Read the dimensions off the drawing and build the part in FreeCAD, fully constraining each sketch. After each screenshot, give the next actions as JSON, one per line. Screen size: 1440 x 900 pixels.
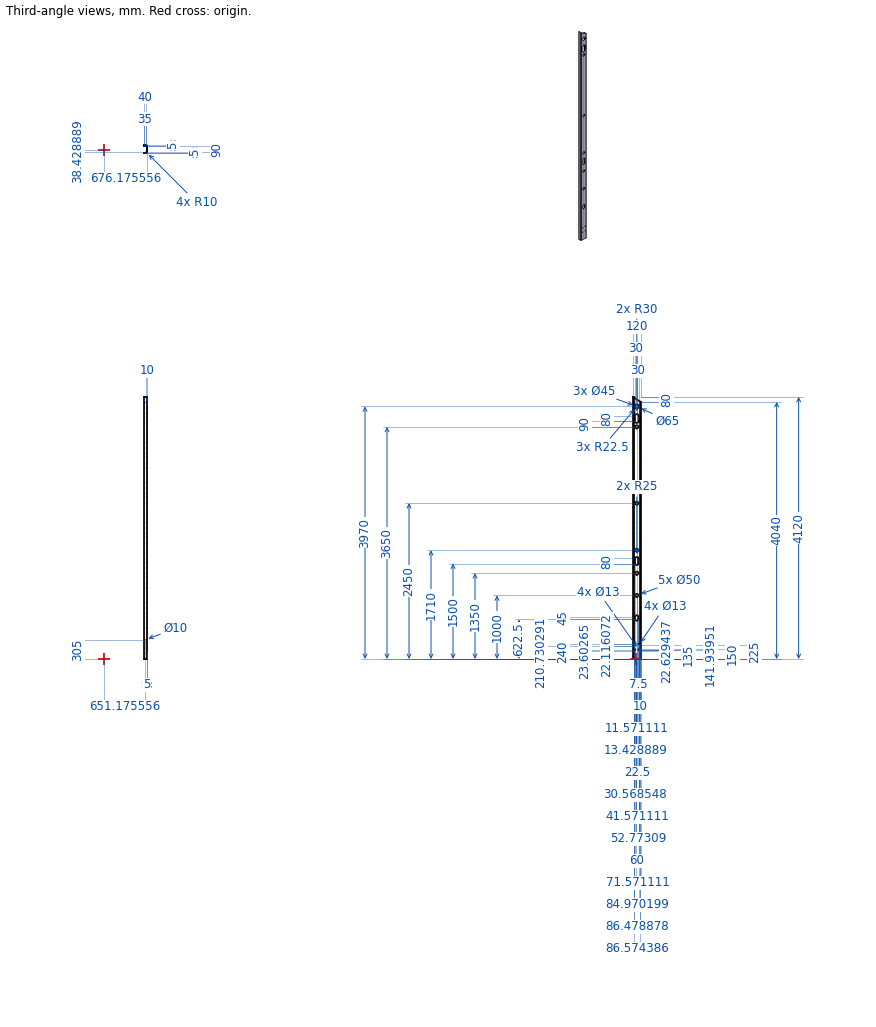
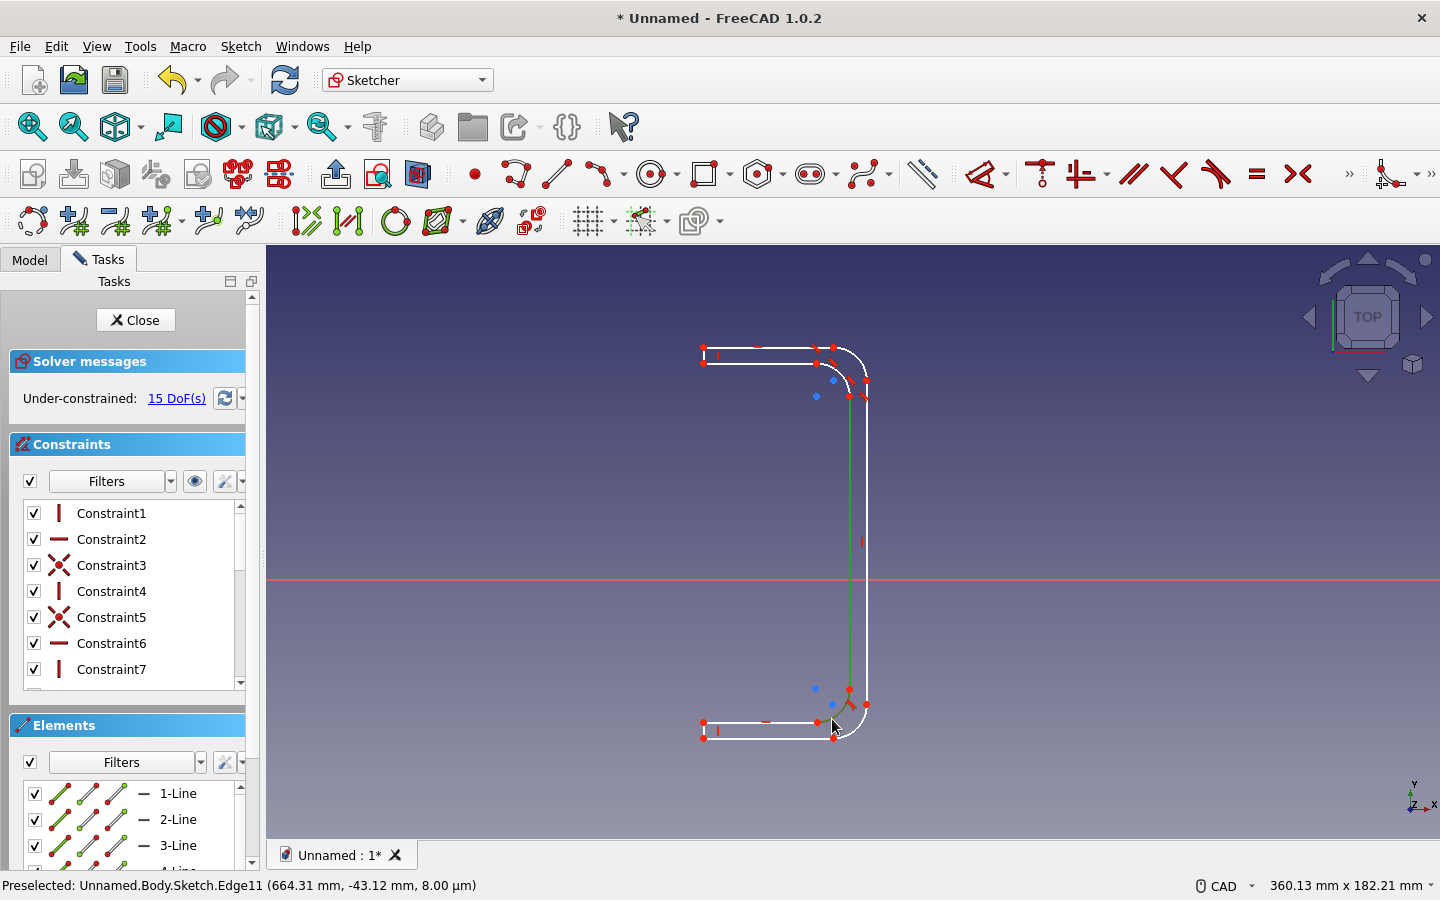
{"action": "left_click", "coordinate": [1216, 174]}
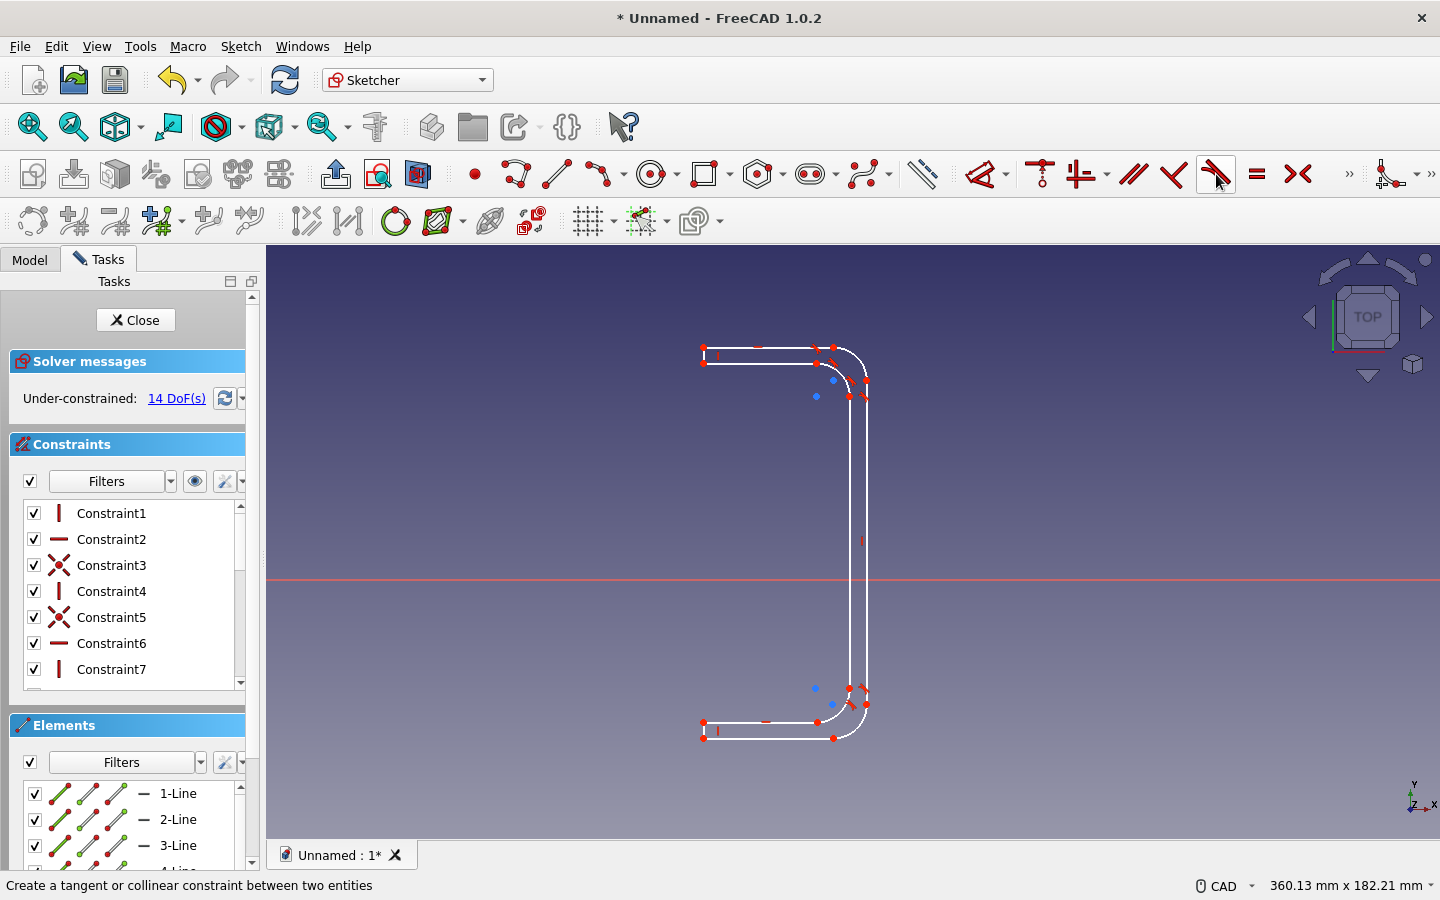
{"action": "left_click", "coordinate": [784, 723]}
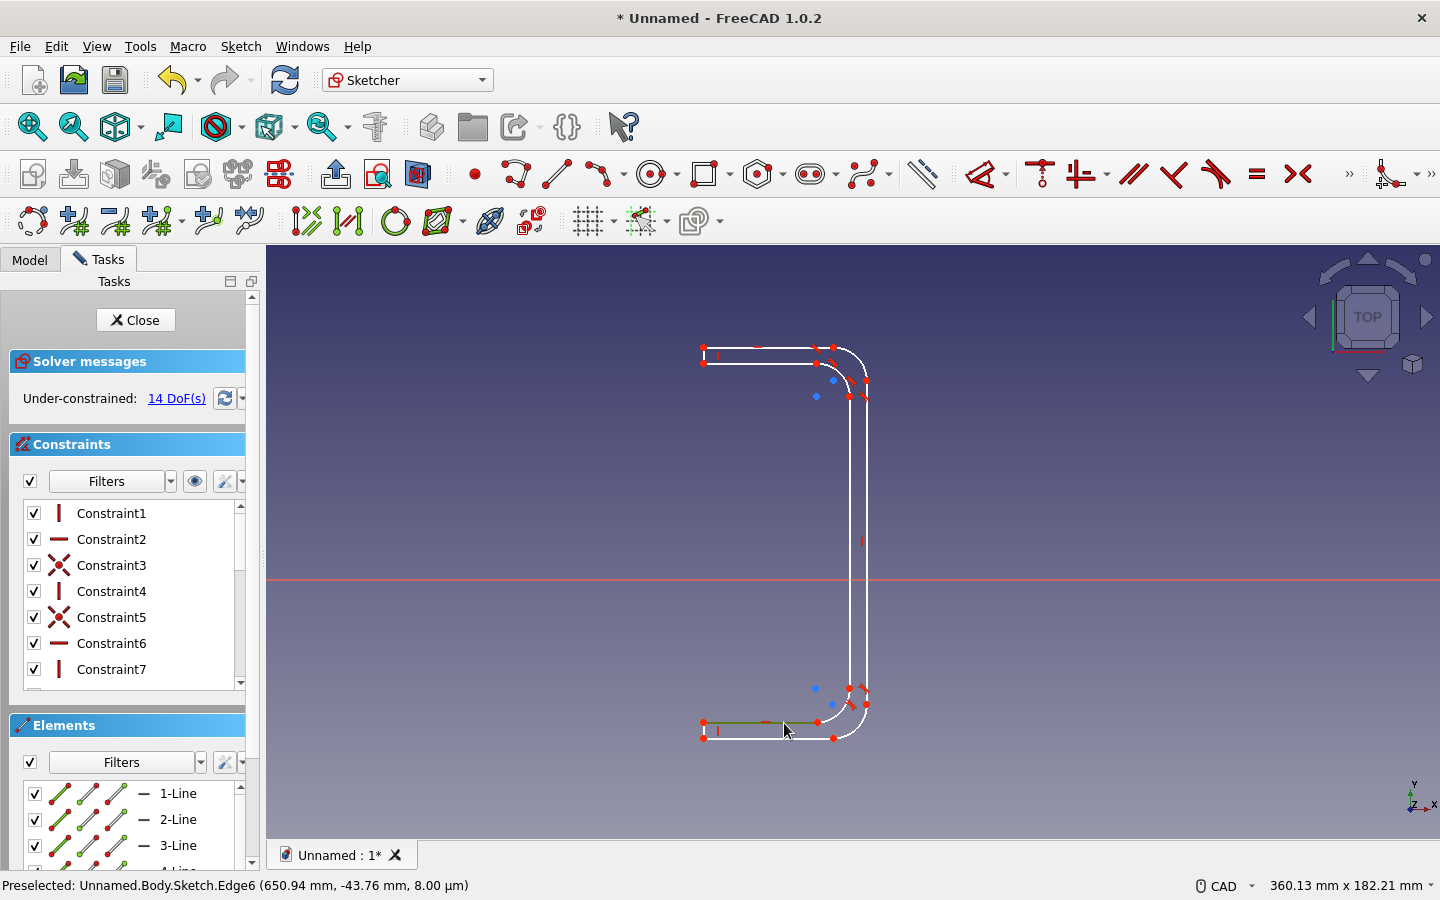
{"action": "left_click", "coordinate": [832, 718]}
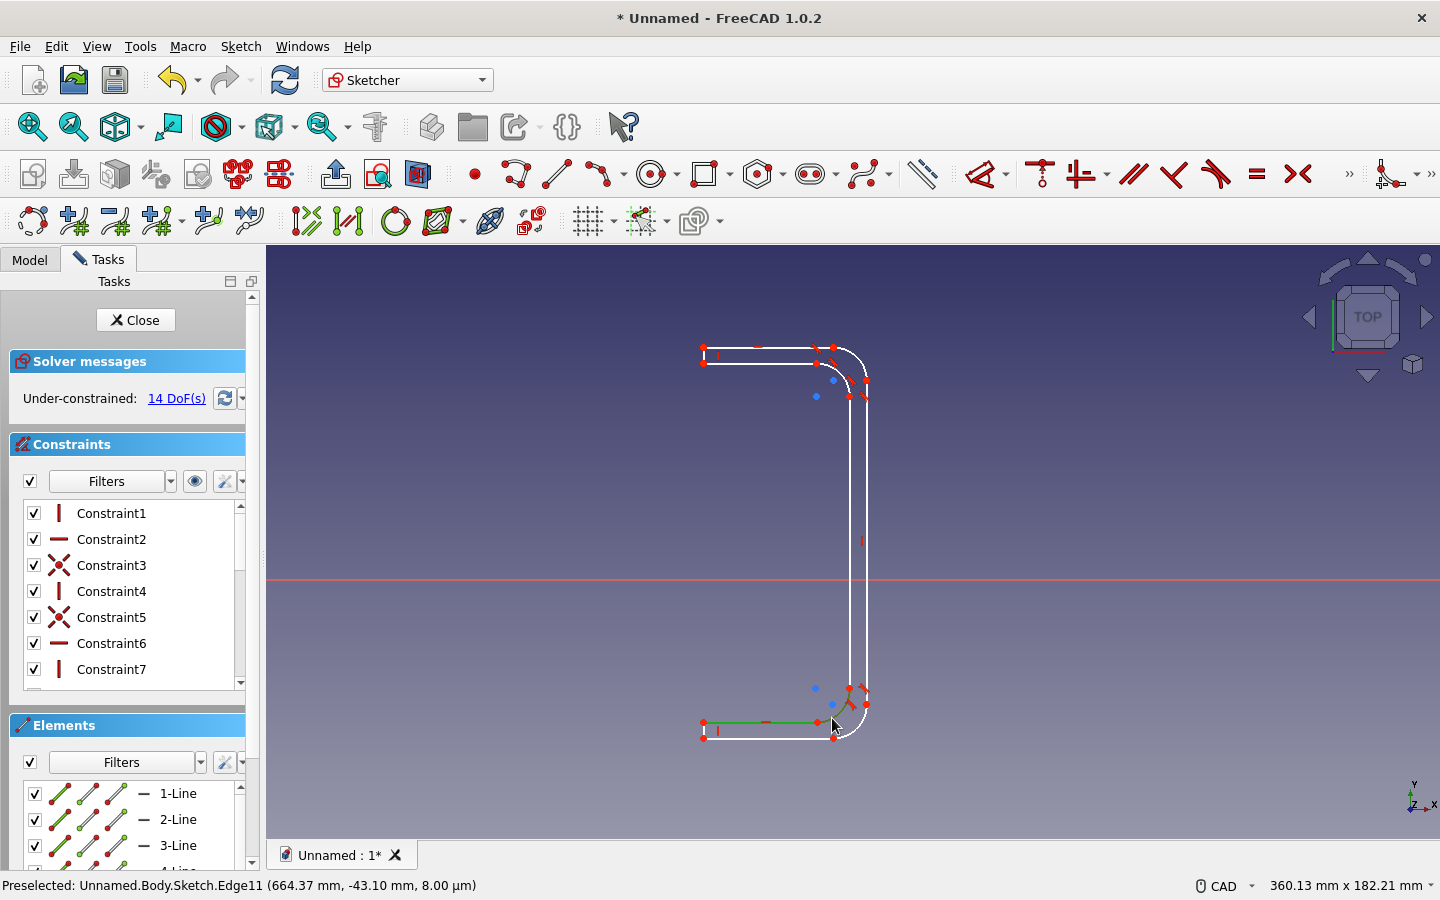
{"action": "key", "text": "t"}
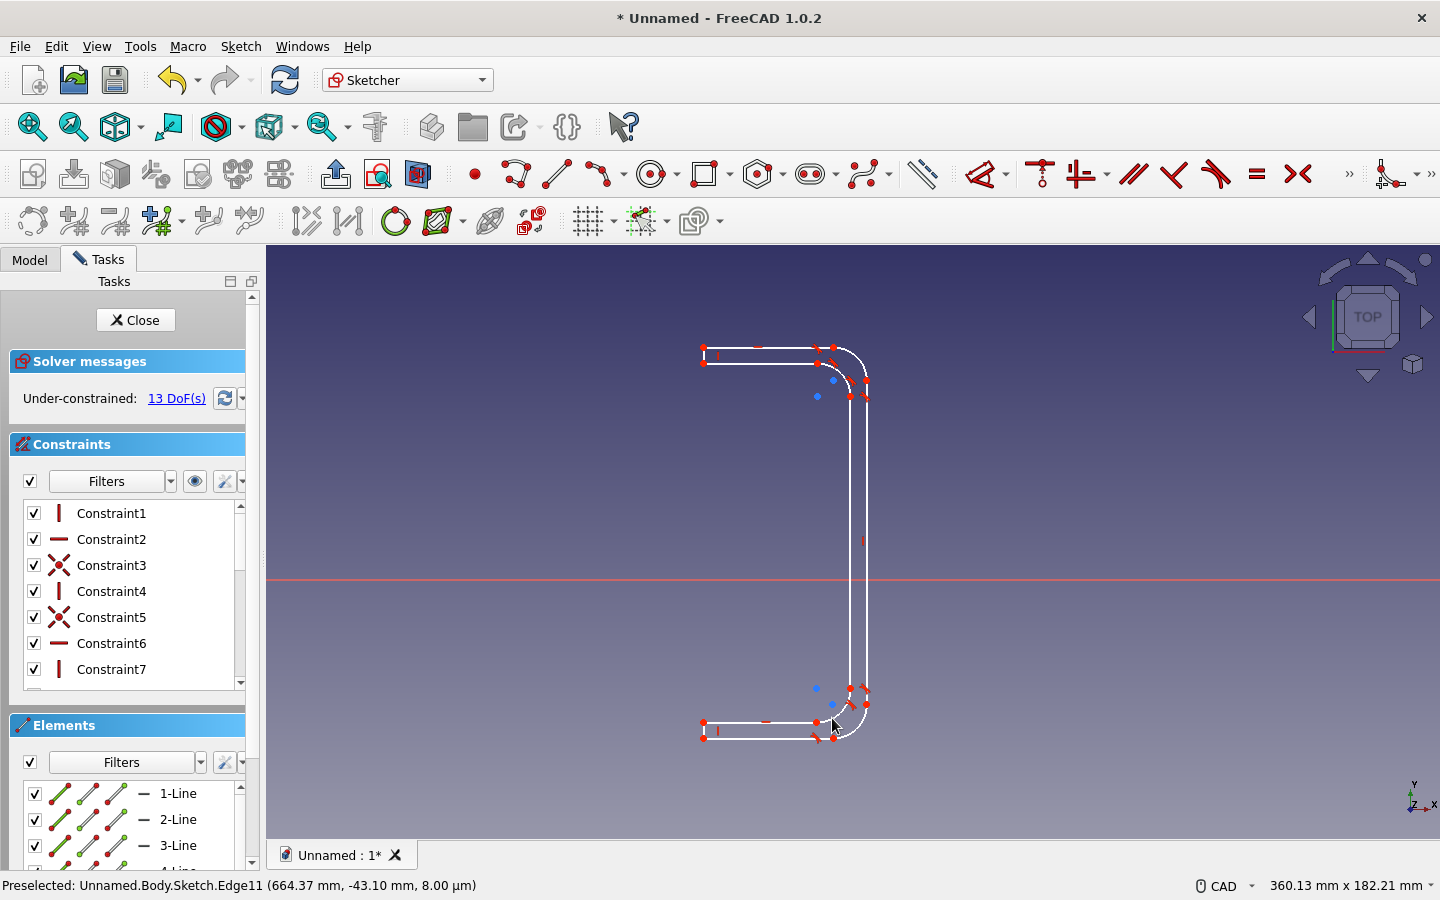
{"action": "left_click", "coordinate": [743, 739]}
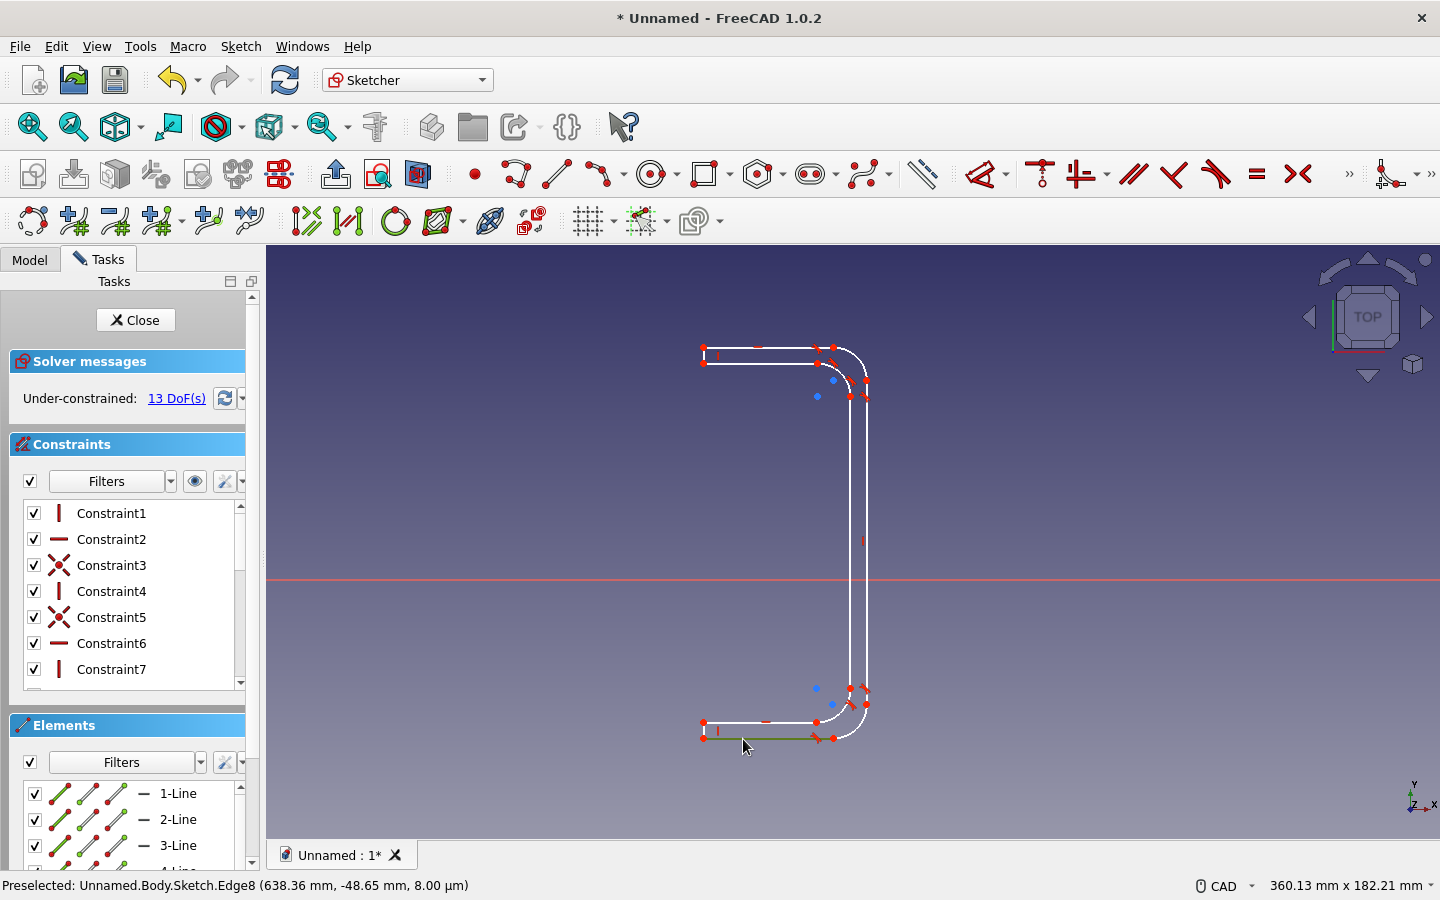
{"action": "left_click", "coordinate": [849, 735]}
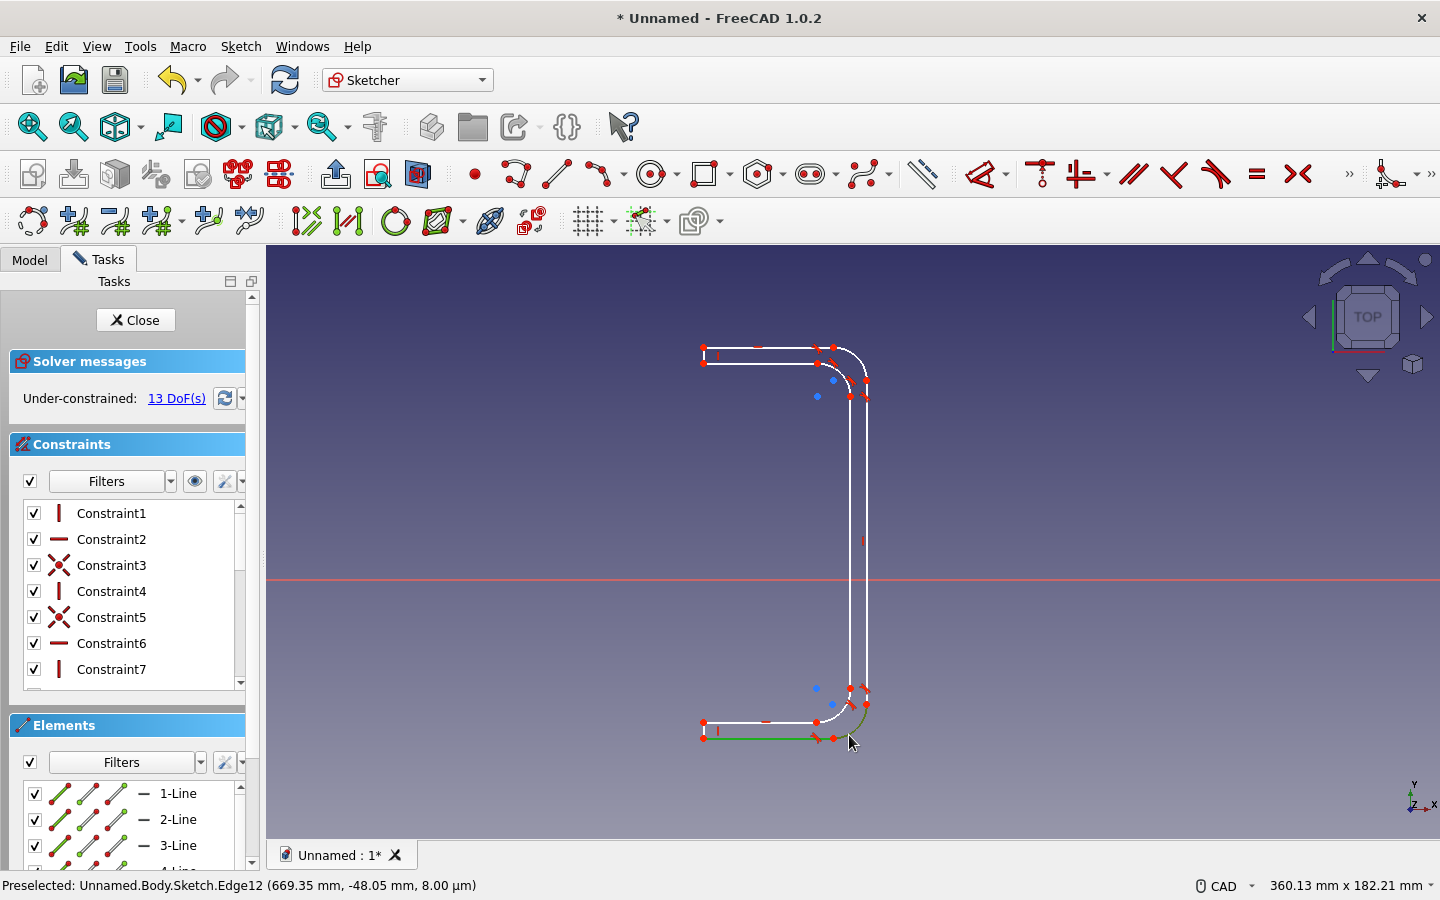
{"action": "key", "text": "t"}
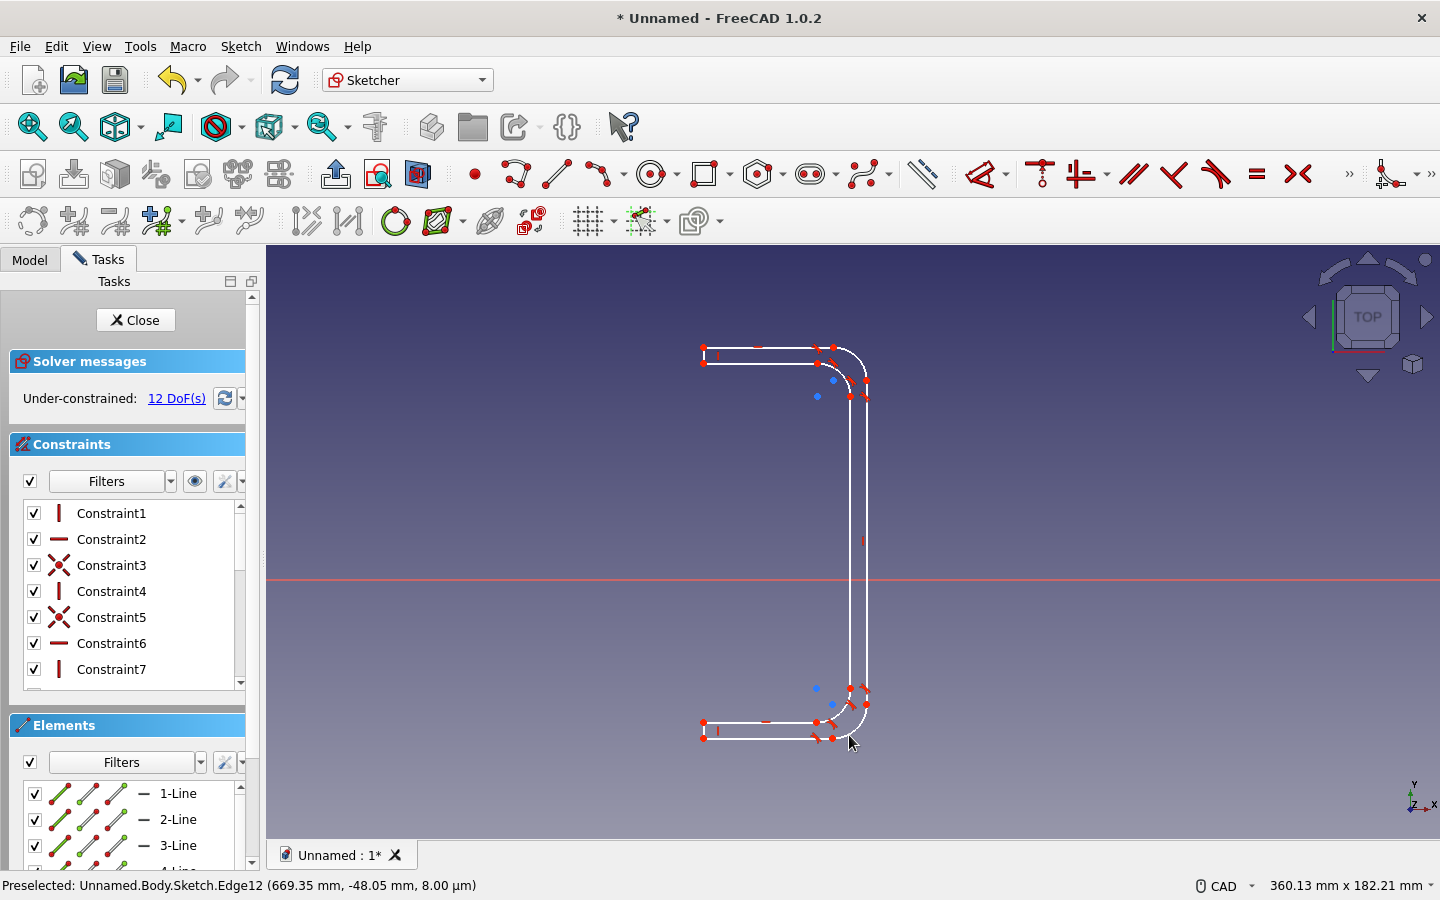
{"action": "left_click", "coordinate": [863, 366]}